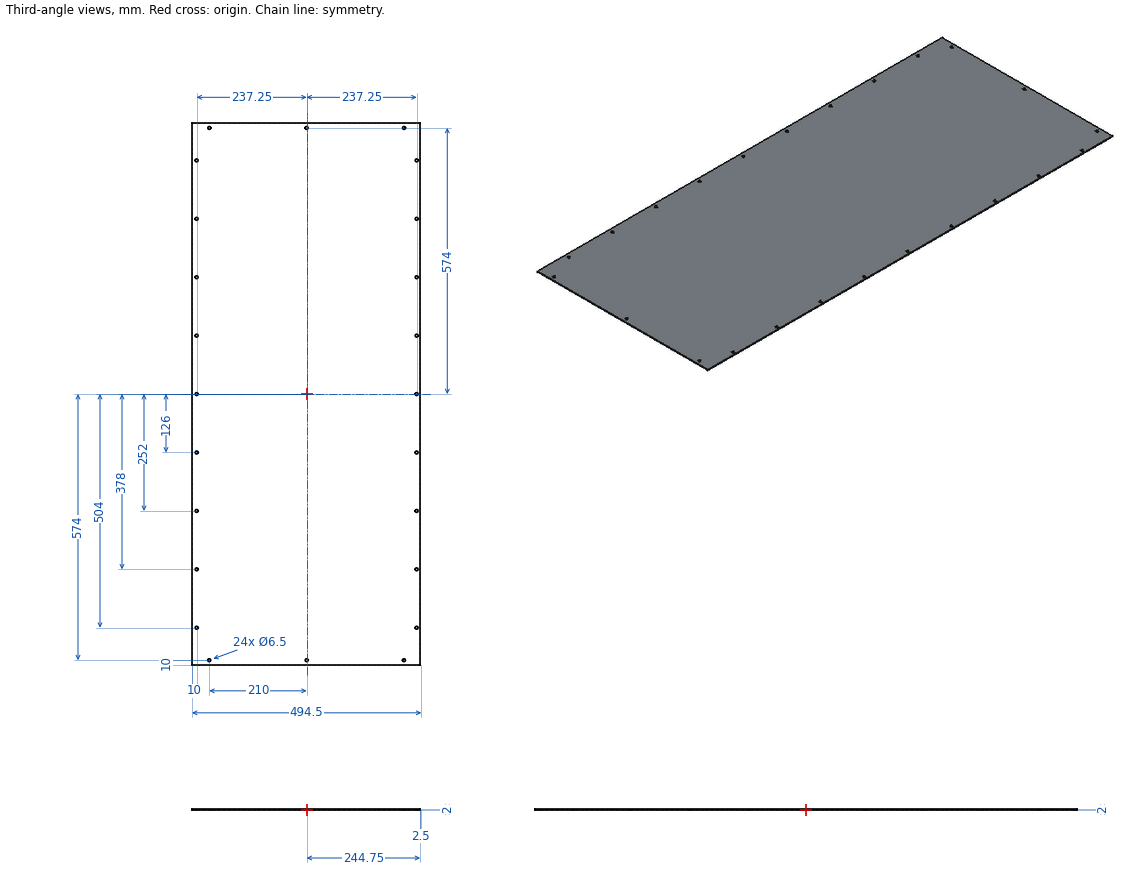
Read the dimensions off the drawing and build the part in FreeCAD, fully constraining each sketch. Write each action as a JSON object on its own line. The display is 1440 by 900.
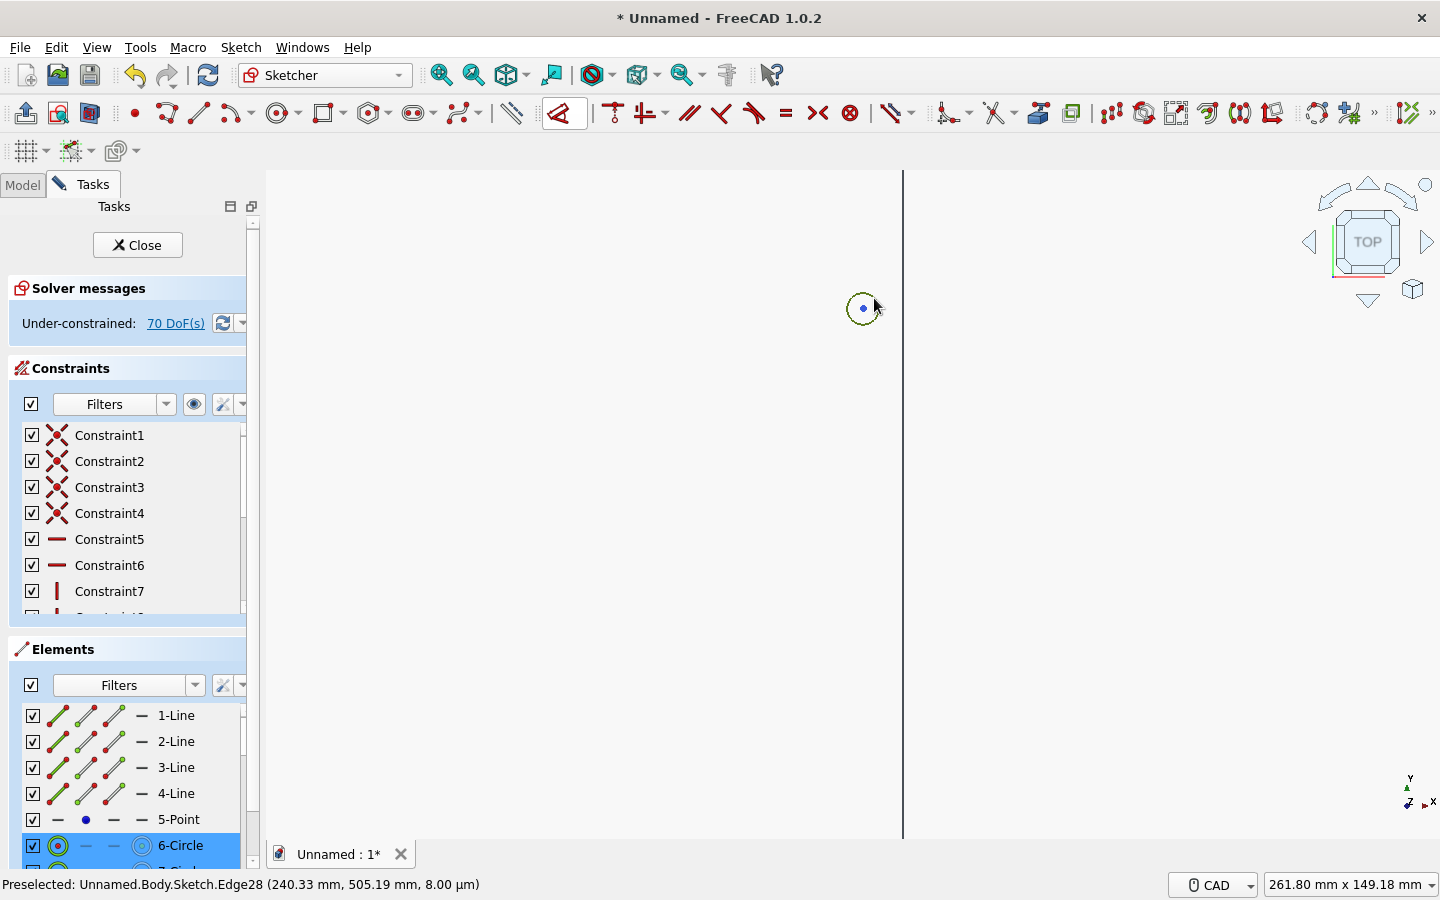
{"action": "scroll", "coordinate": [883, 299], "scroll_direction": "down", "scroll_amount": 12}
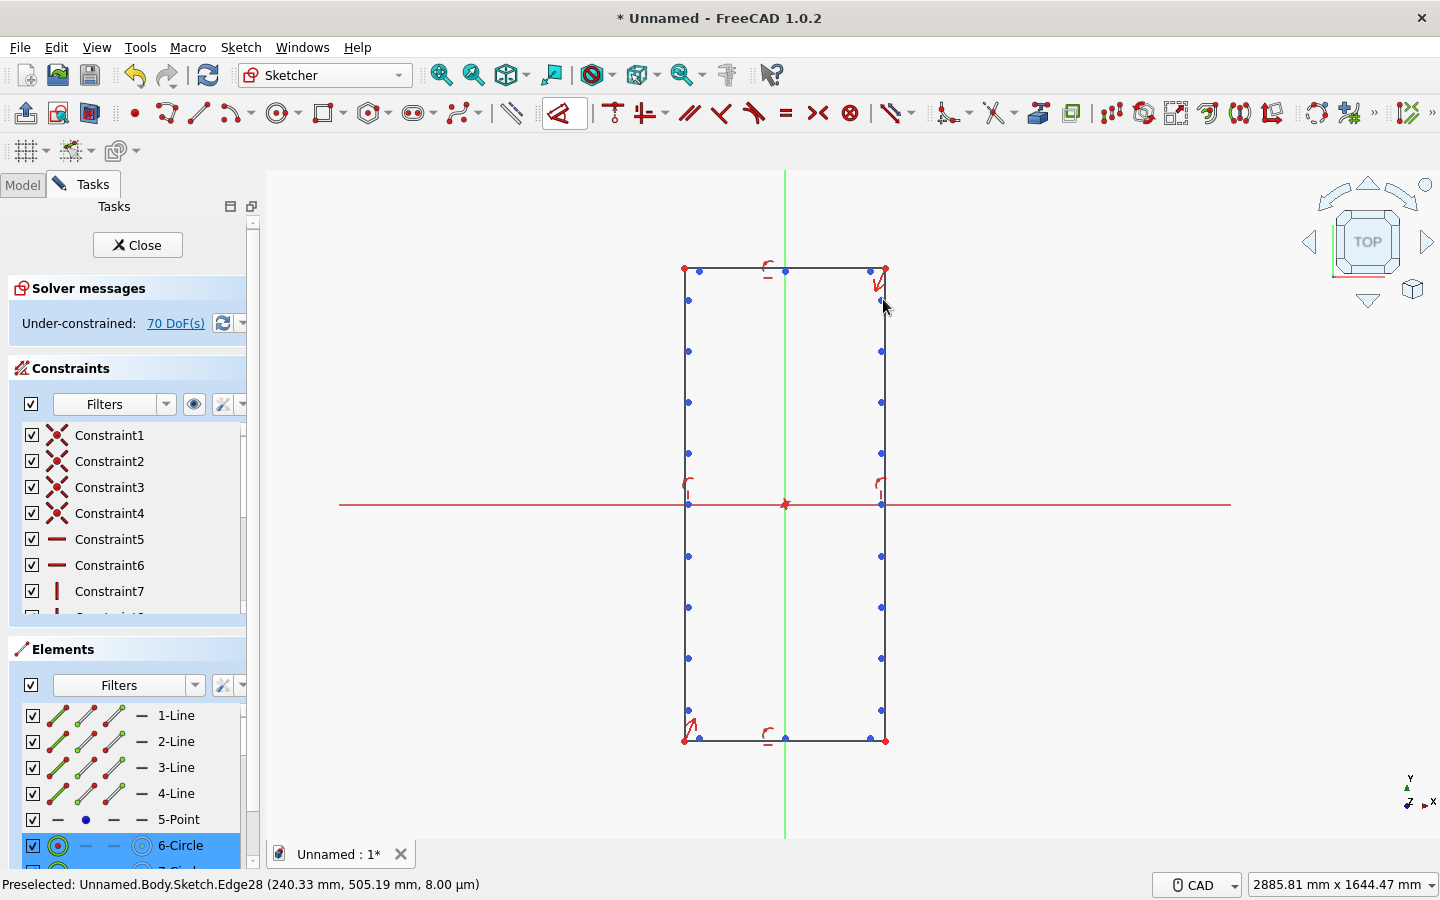
{"action": "scroll", "coordinate": [871, 271], "scroll_direction": "up", "scroll_amount": 12}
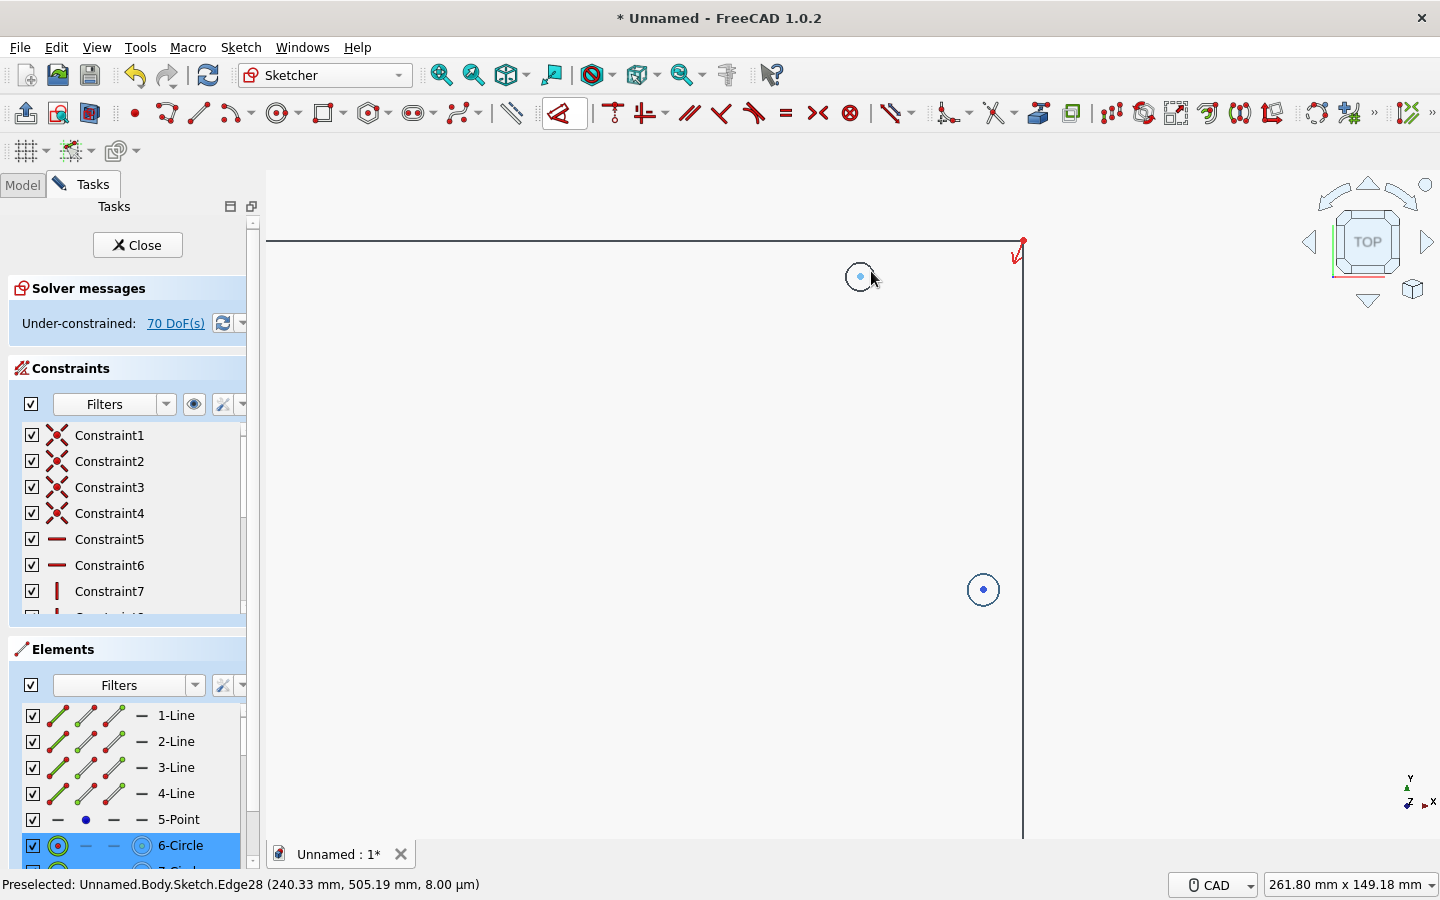
{"action": "left_click", "coordinate": [870, 267]}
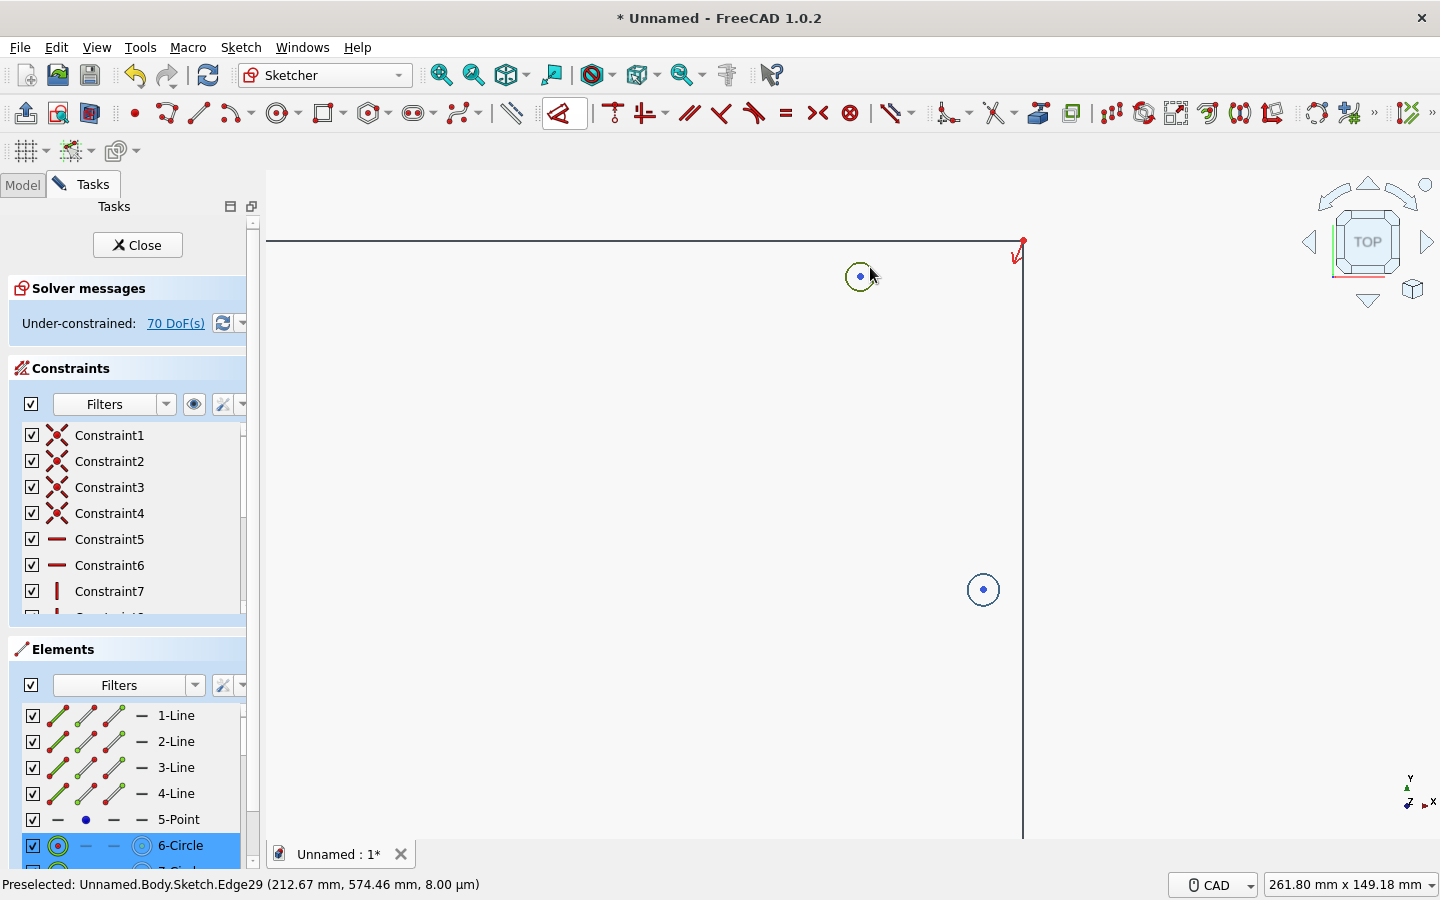
{"action": "left_click", "coordinate": [786, 114]}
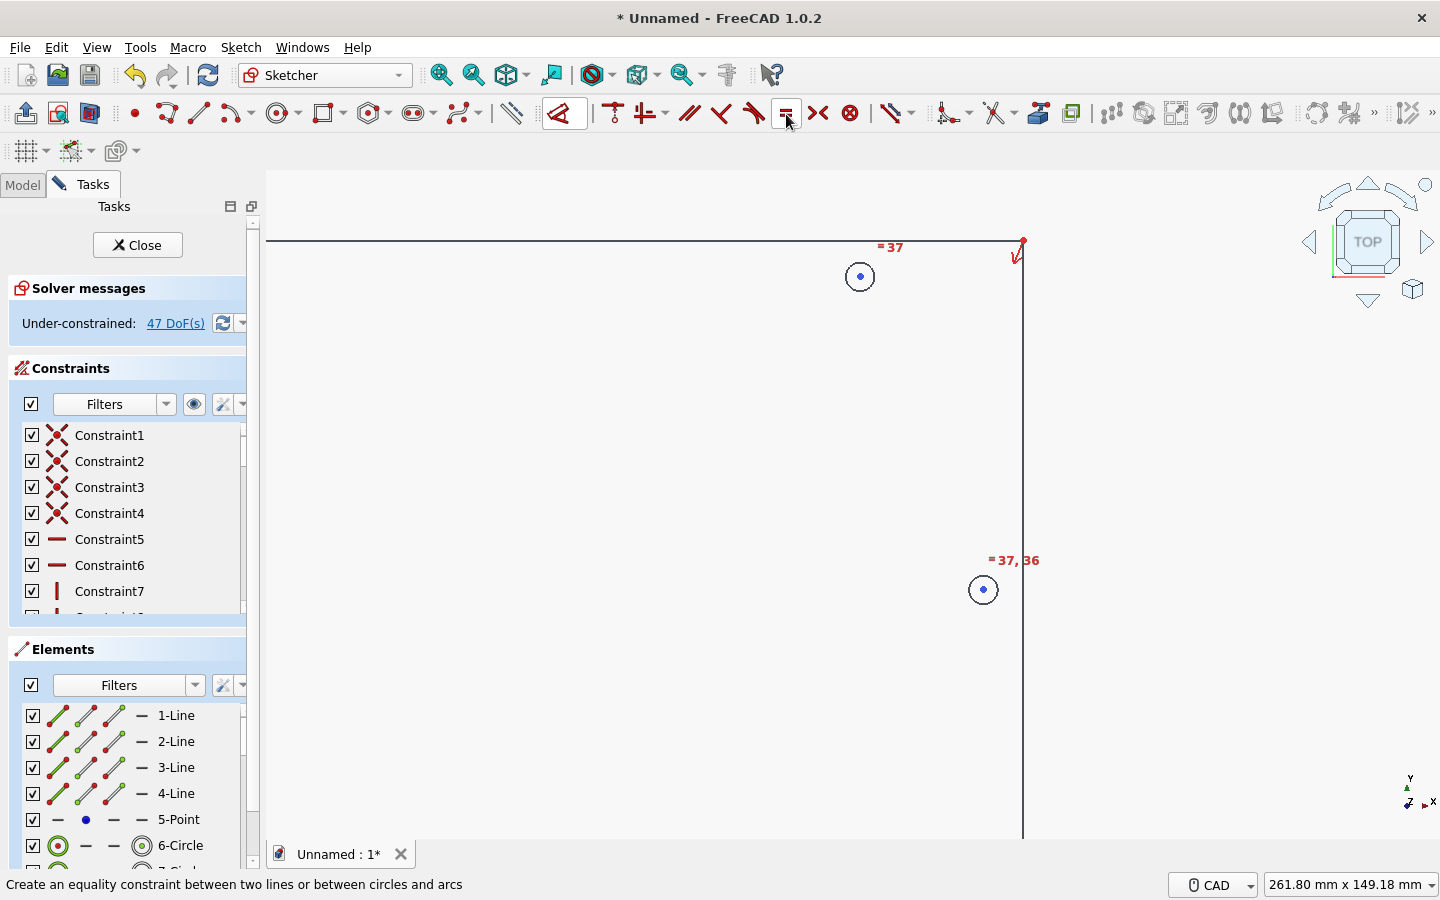
{"action": "scroll", "coordinate": [871, 271], "scroll_direction": "down", "scroll_amount": 12}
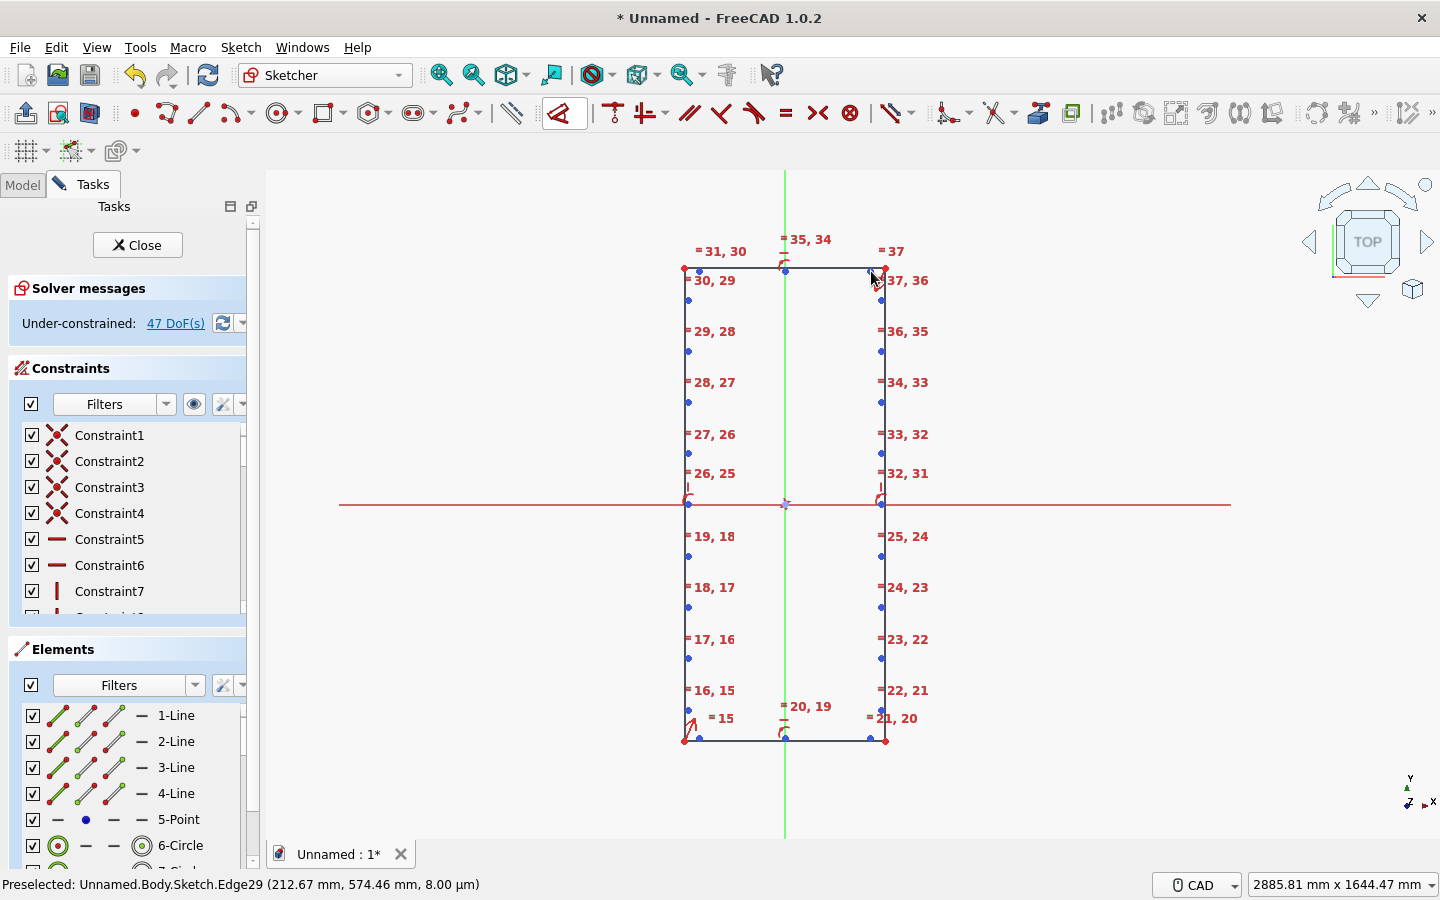
{"action": "left_click", "coordinate": [700, 739]}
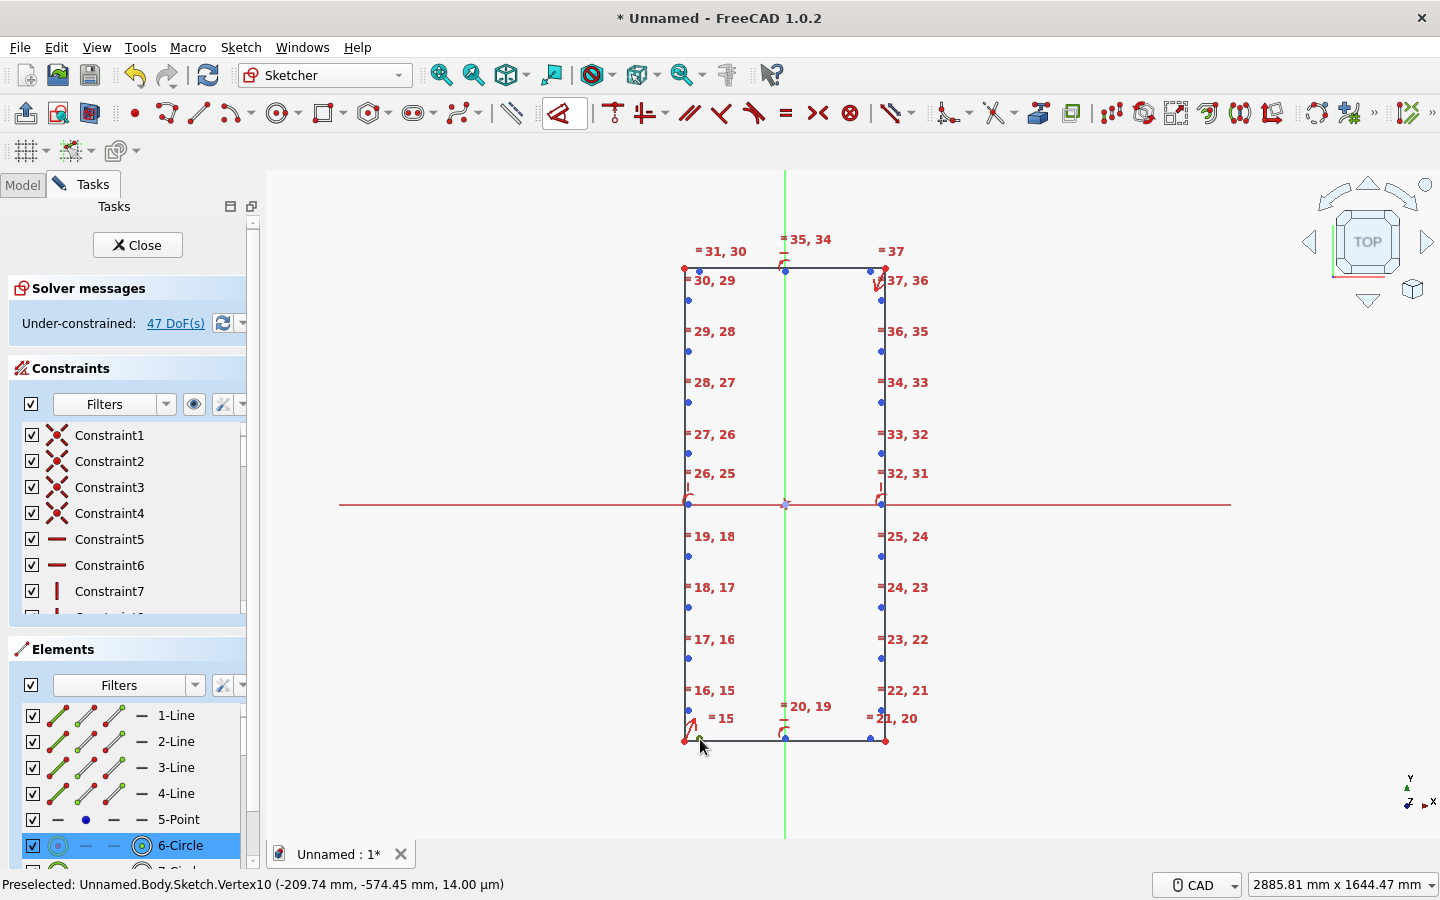
{"action": "left_click", "coordinate": [871, 739]}